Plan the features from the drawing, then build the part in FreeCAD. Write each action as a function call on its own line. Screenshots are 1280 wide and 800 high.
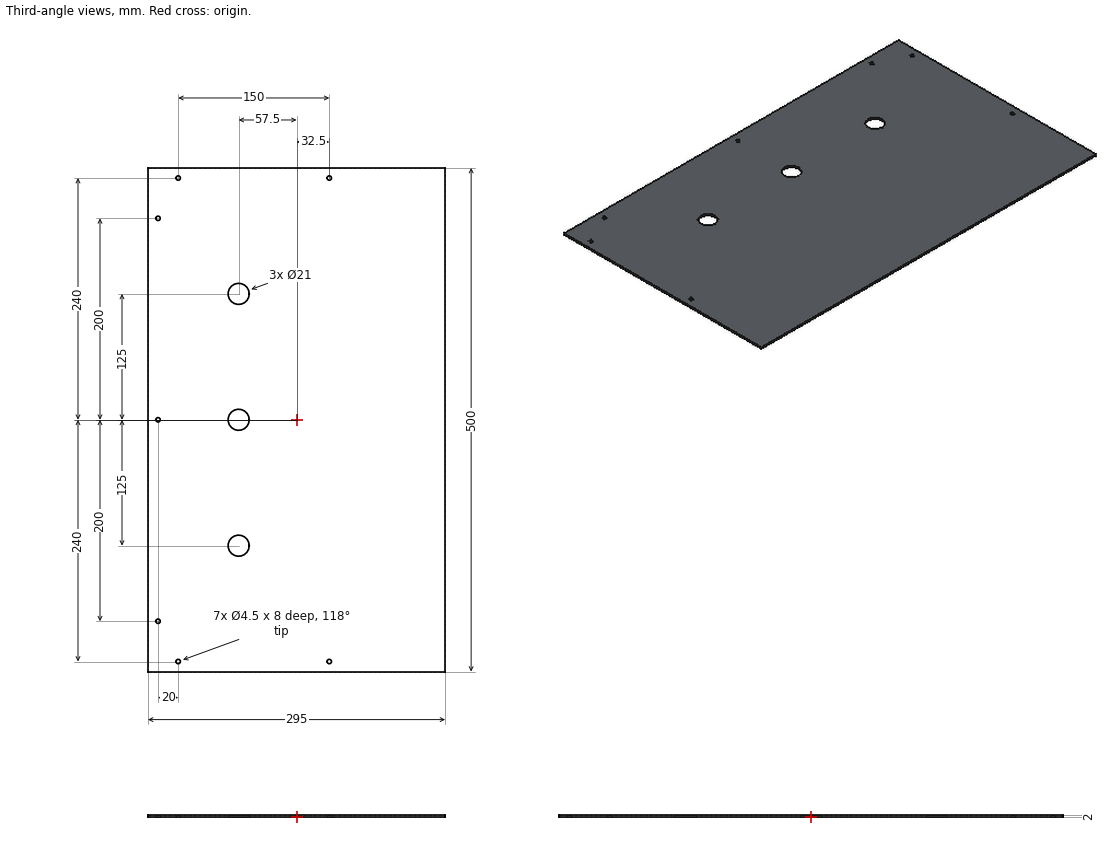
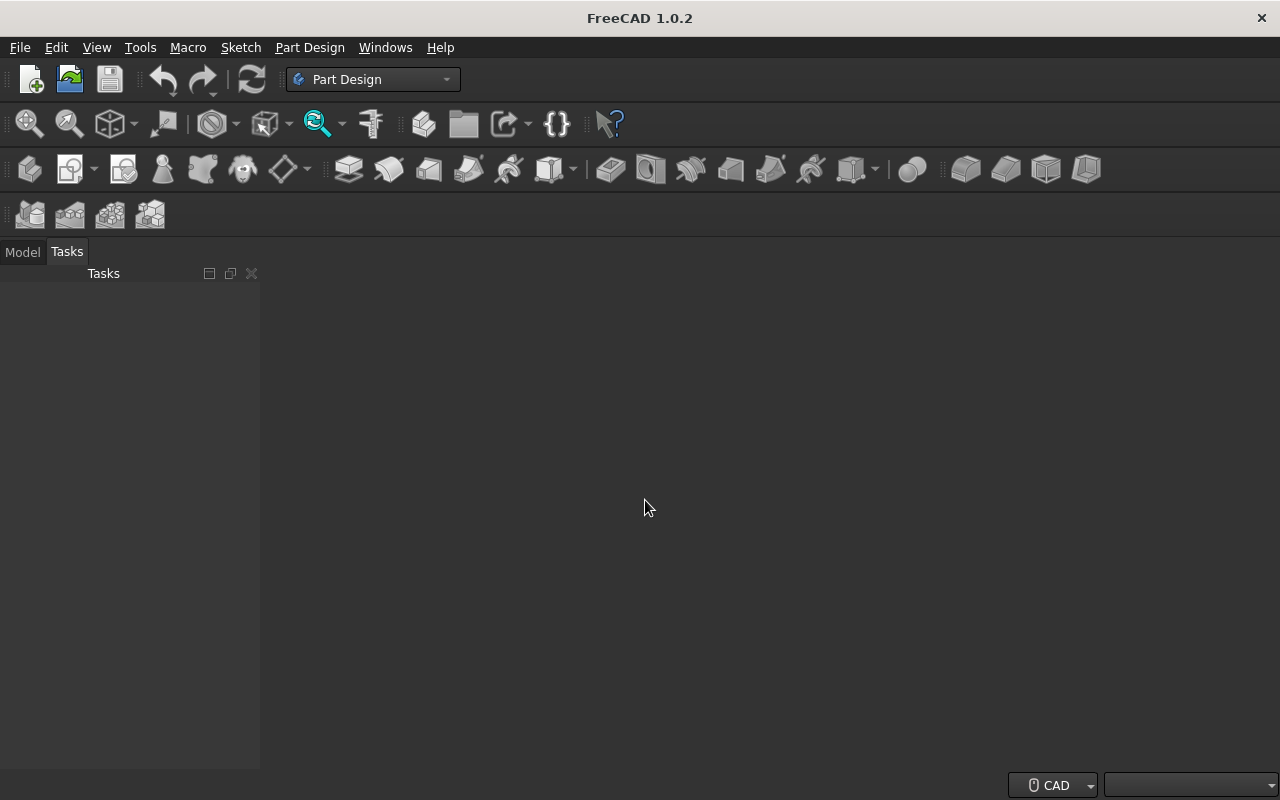
key(ctrl+n)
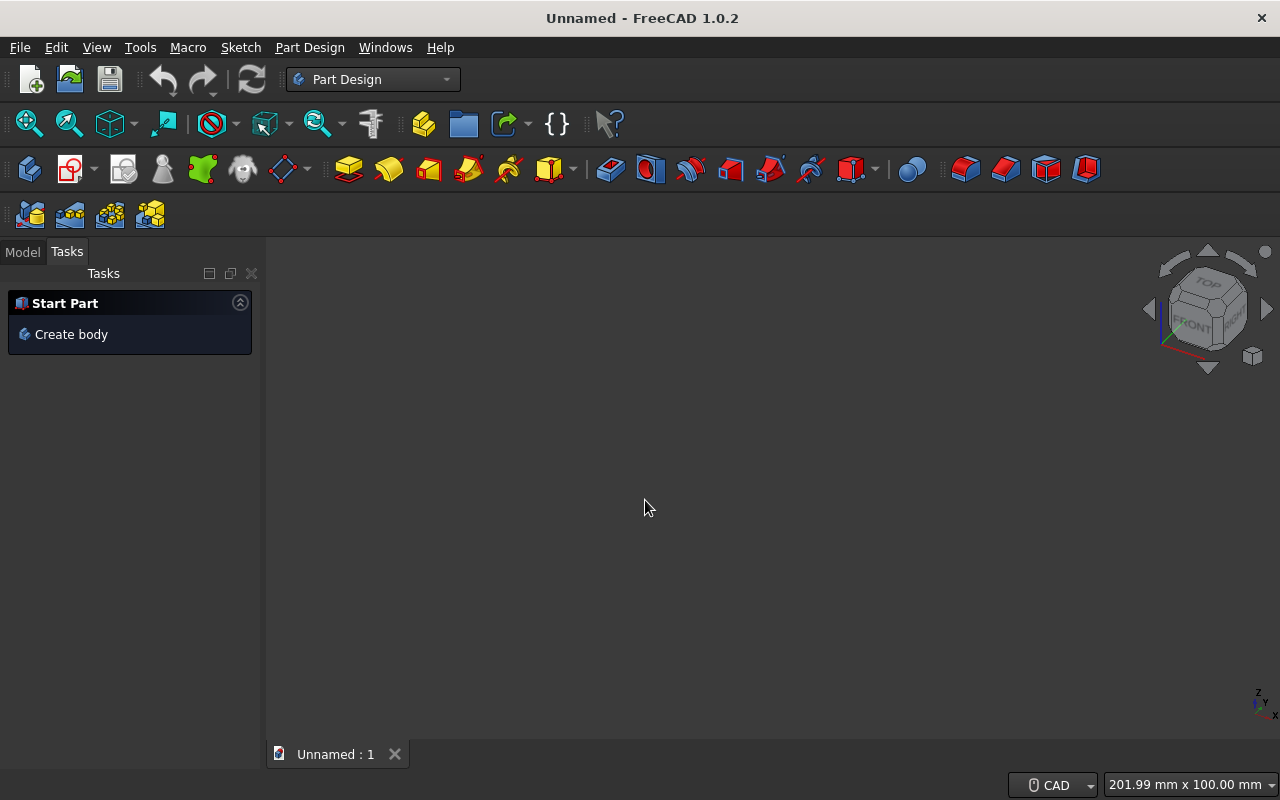
click(70, 170)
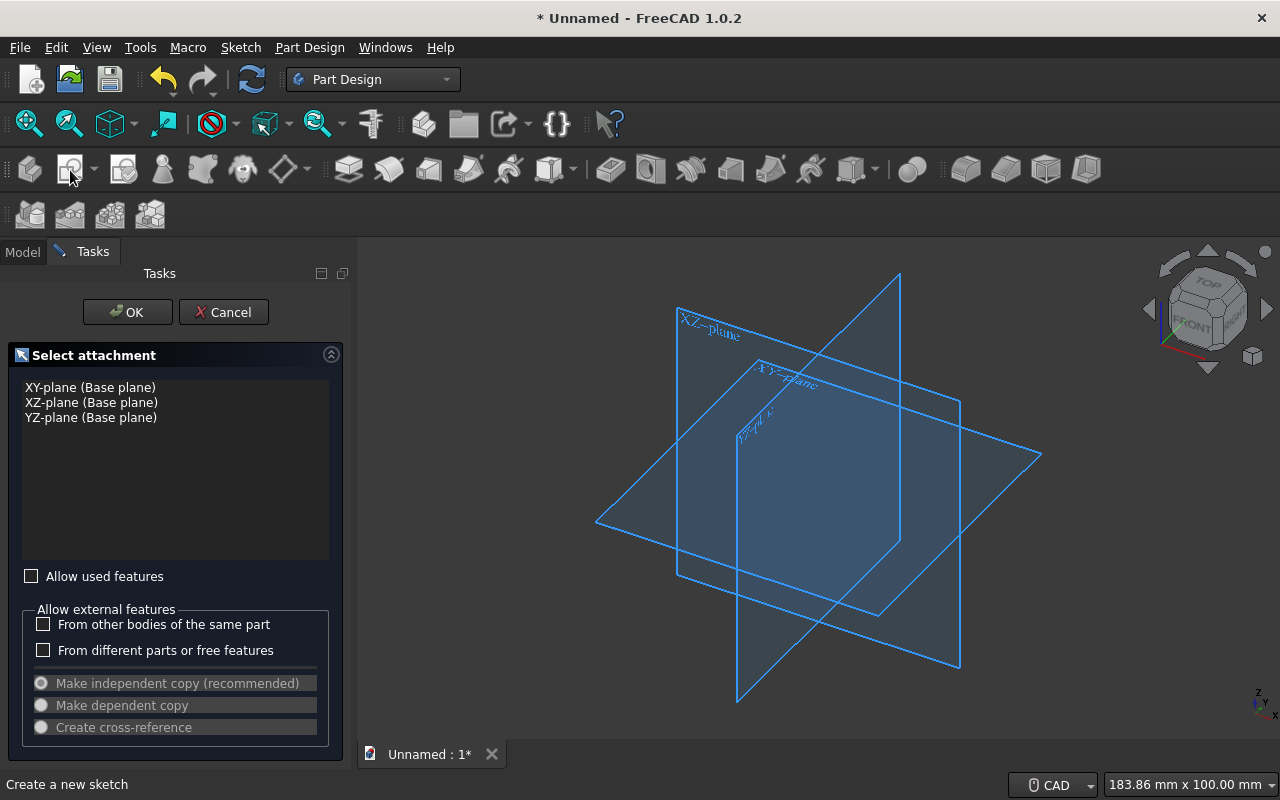
click(82, 388)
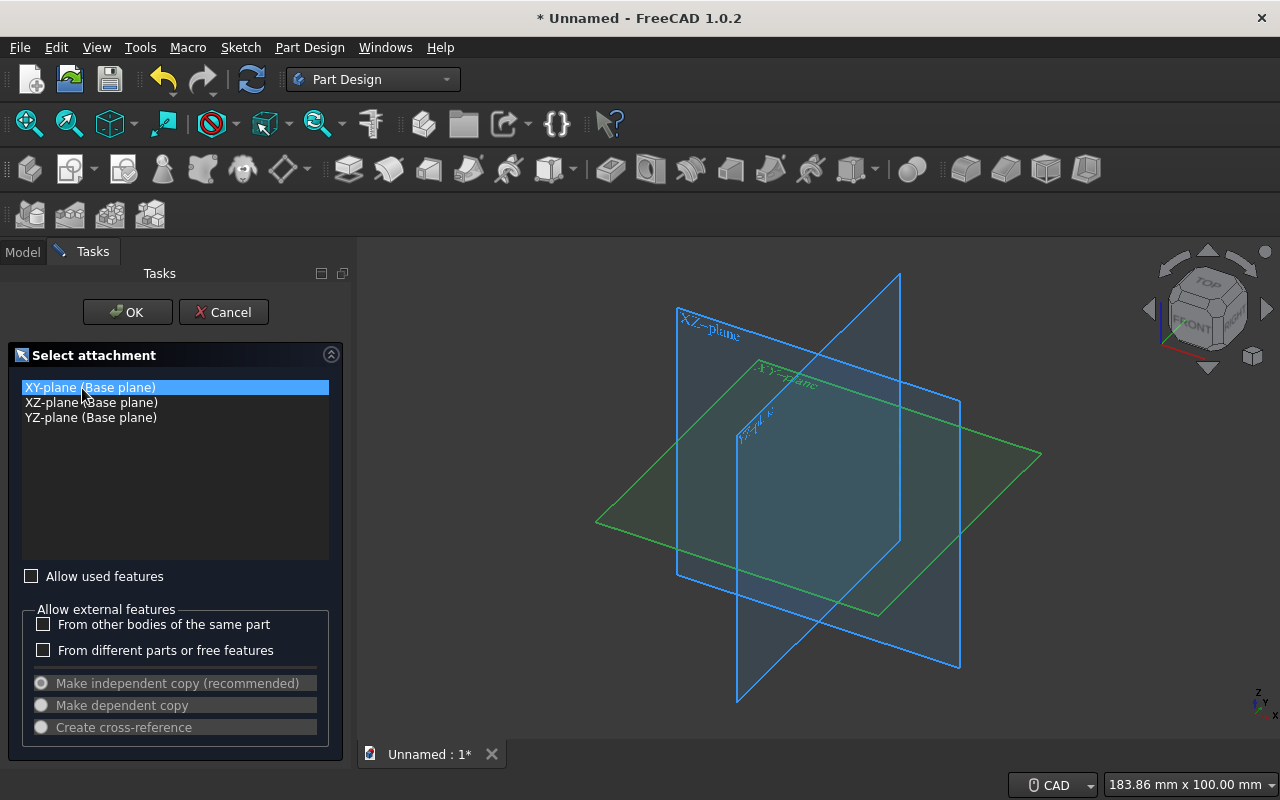
click(128, 312)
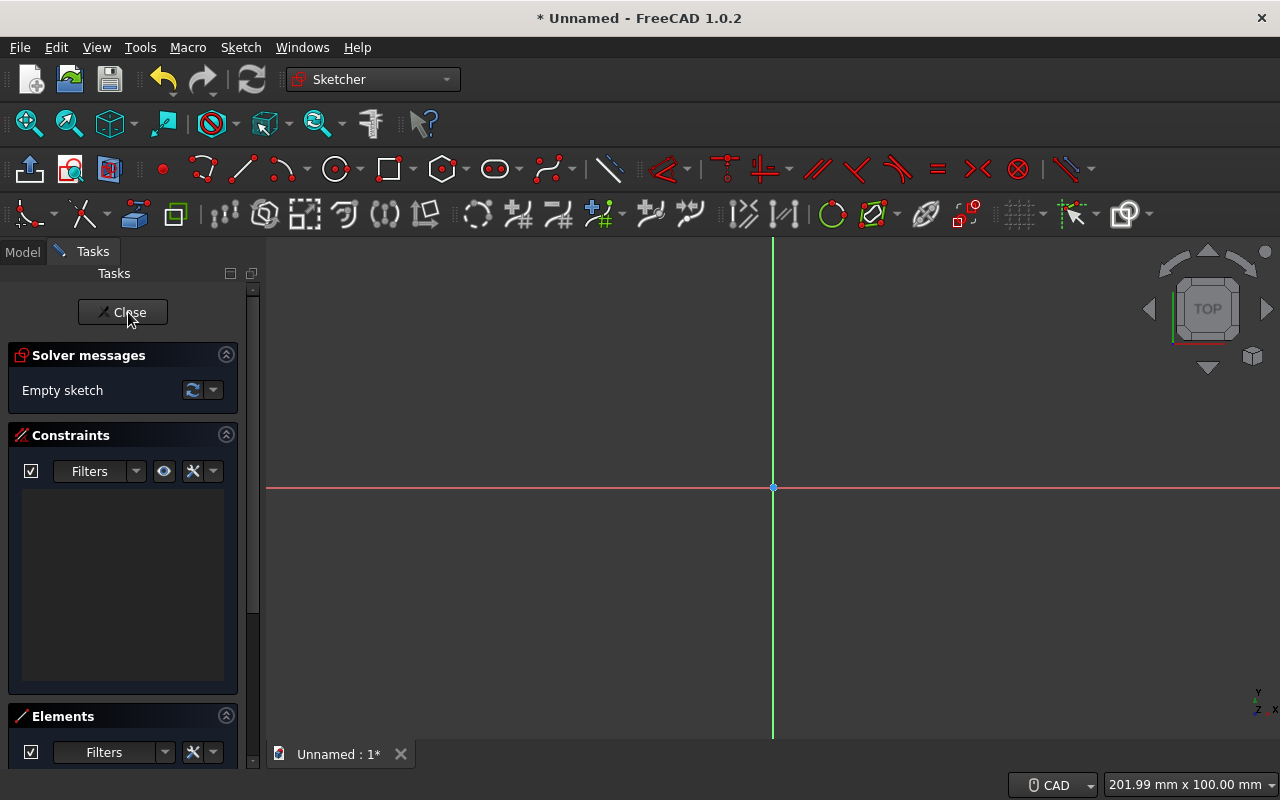
scroll(694, 488, down, 10)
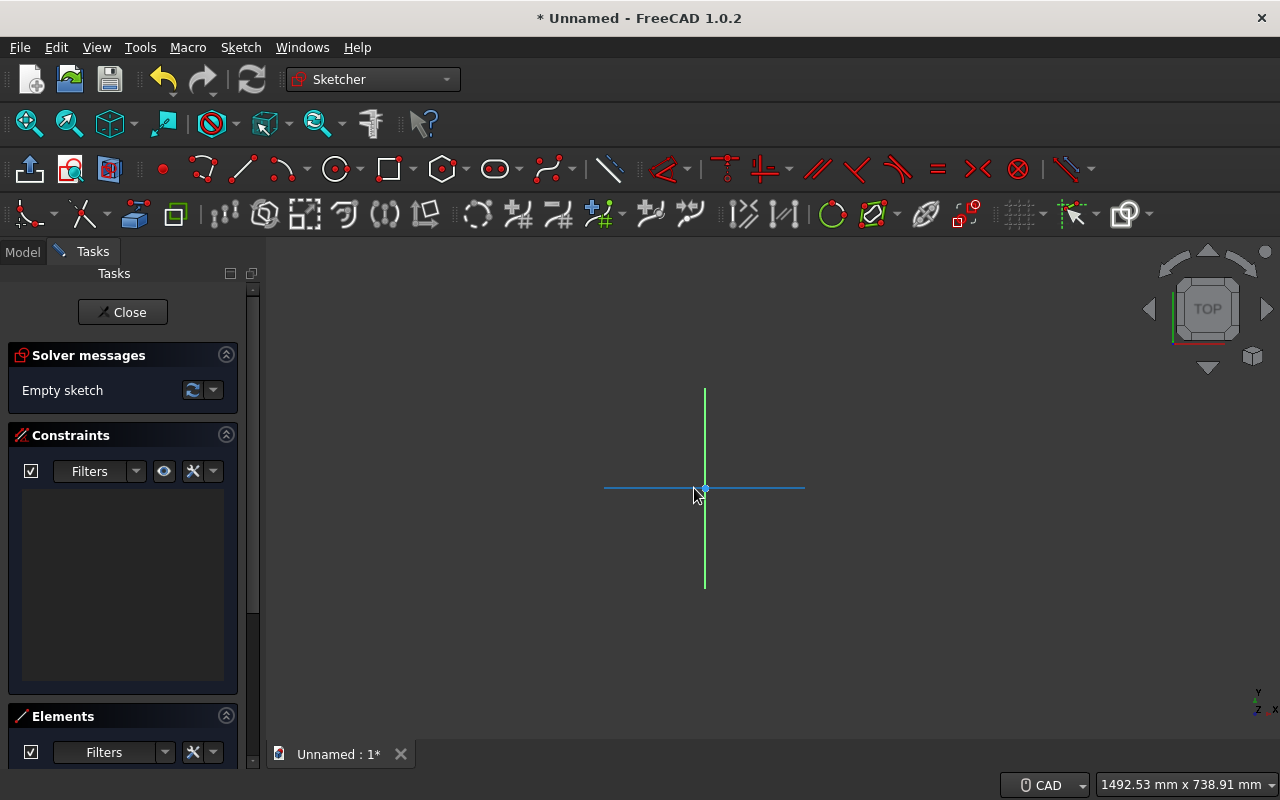
click(416, 170)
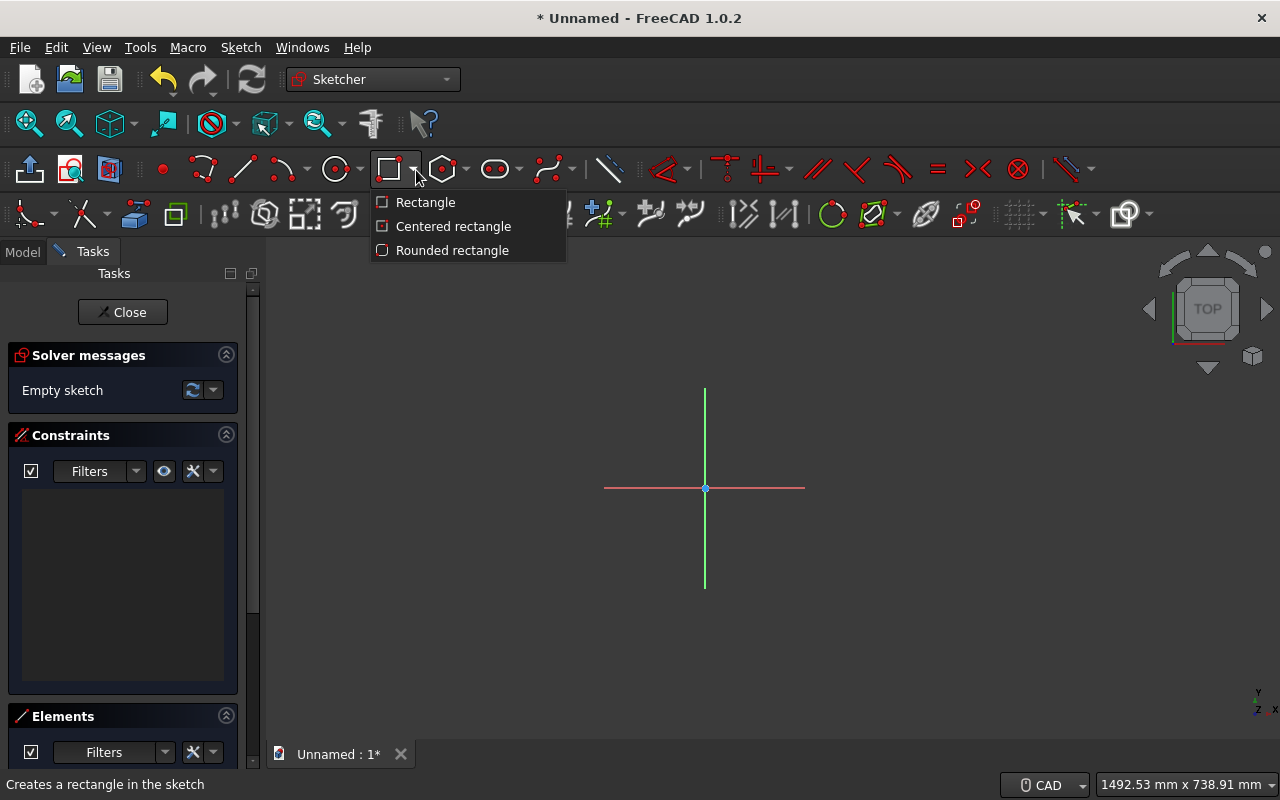
click(468, 226)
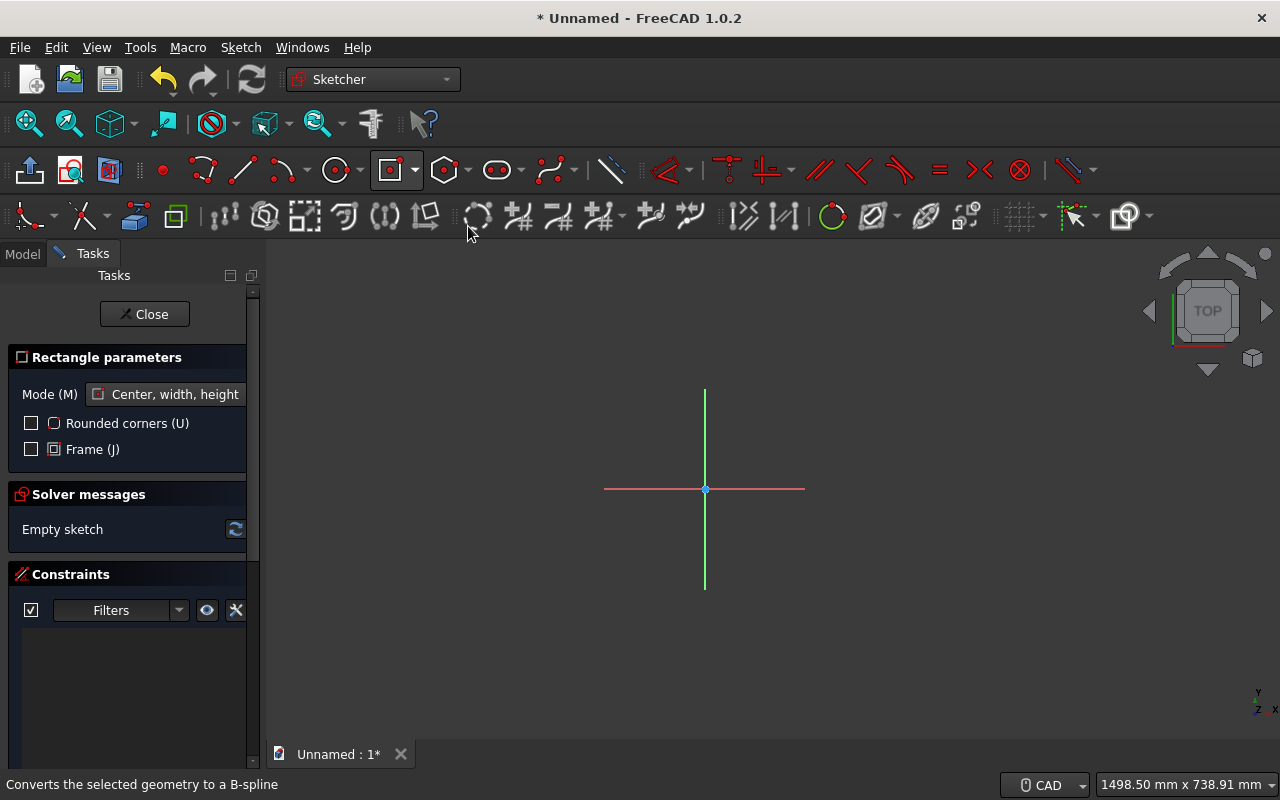
click(705, 489)
move(805, 320)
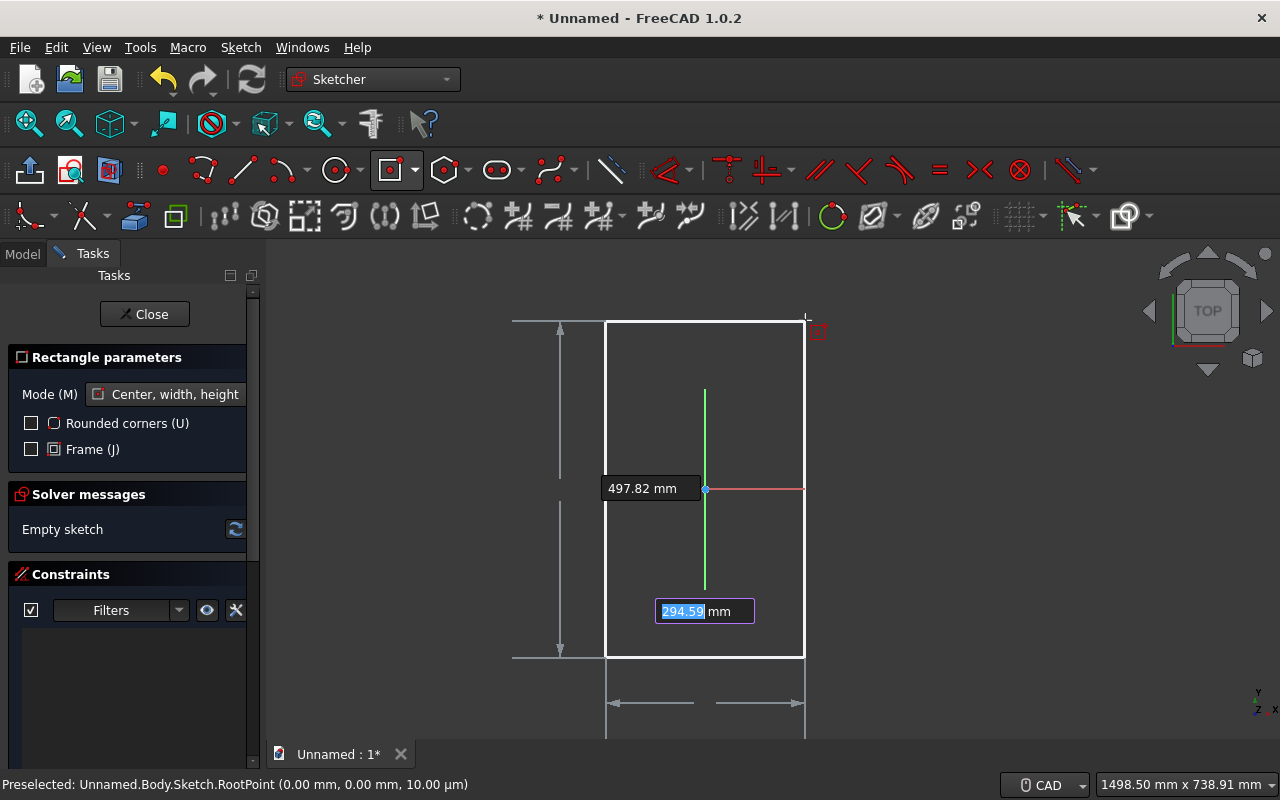
text(295)
key(Tab)
text(500)
key(Return)
key(Escape)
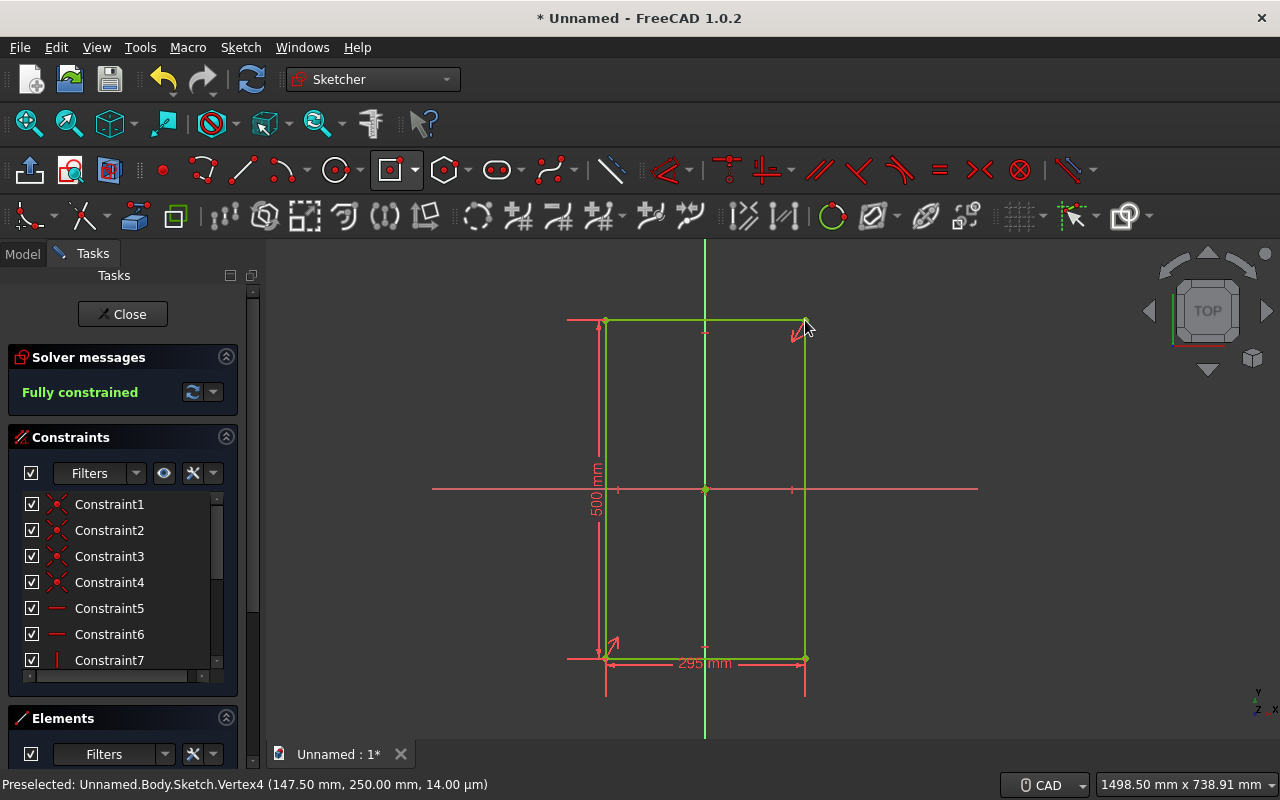
click(123, 314)